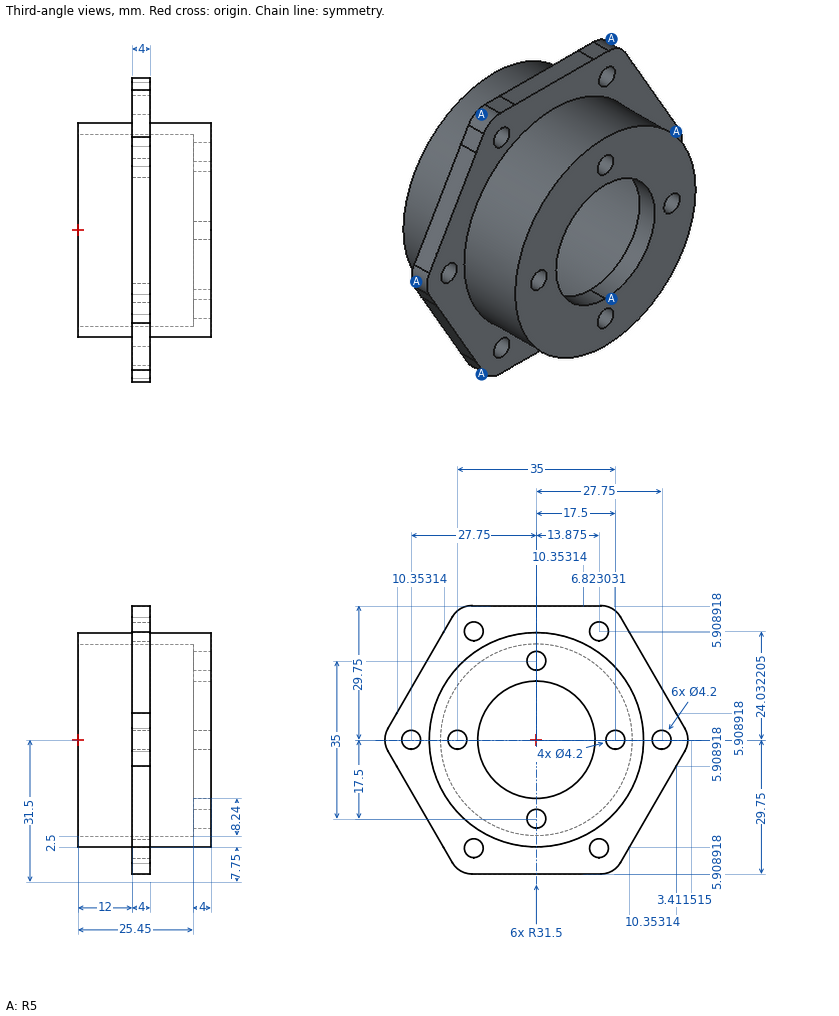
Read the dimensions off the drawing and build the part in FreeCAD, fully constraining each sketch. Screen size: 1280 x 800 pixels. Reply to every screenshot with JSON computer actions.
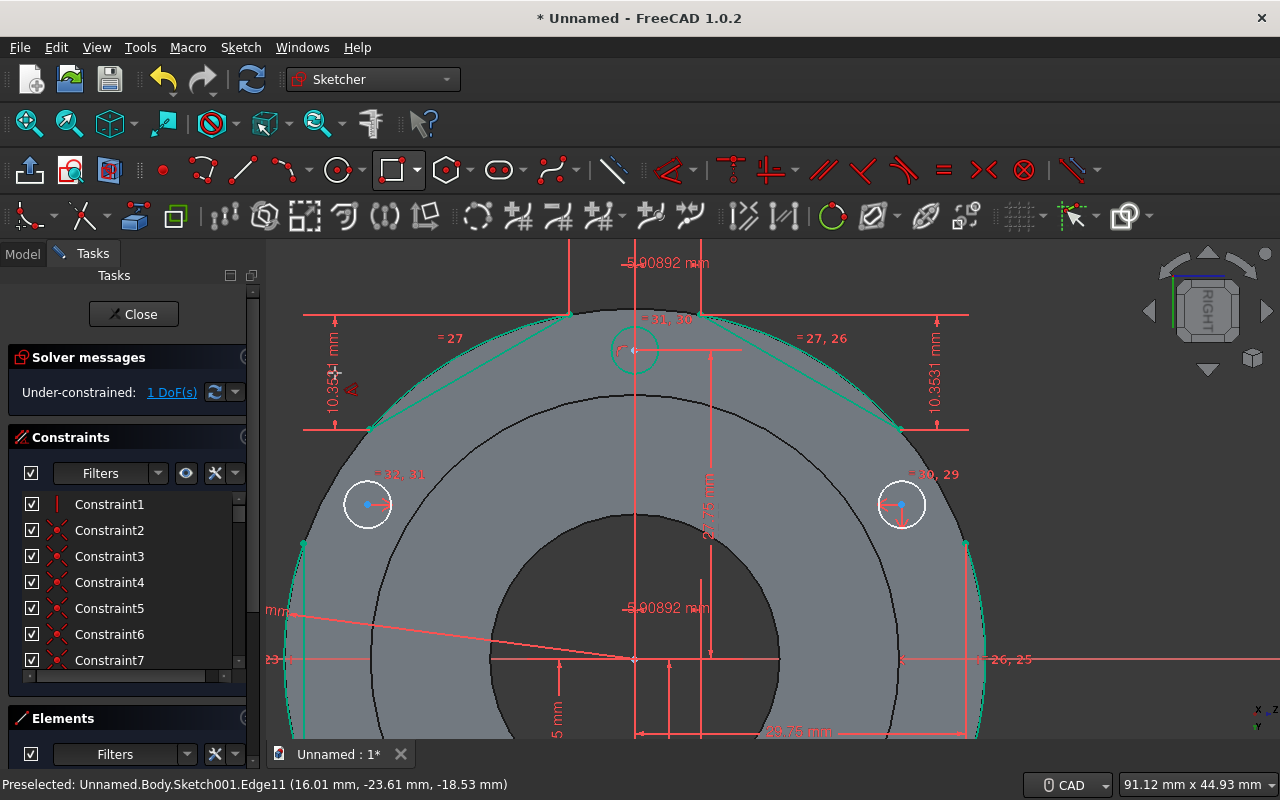
{"action": "scroll", "coordinate": [761, 350], "scroll_direction": "down", "scroll_amount": 4}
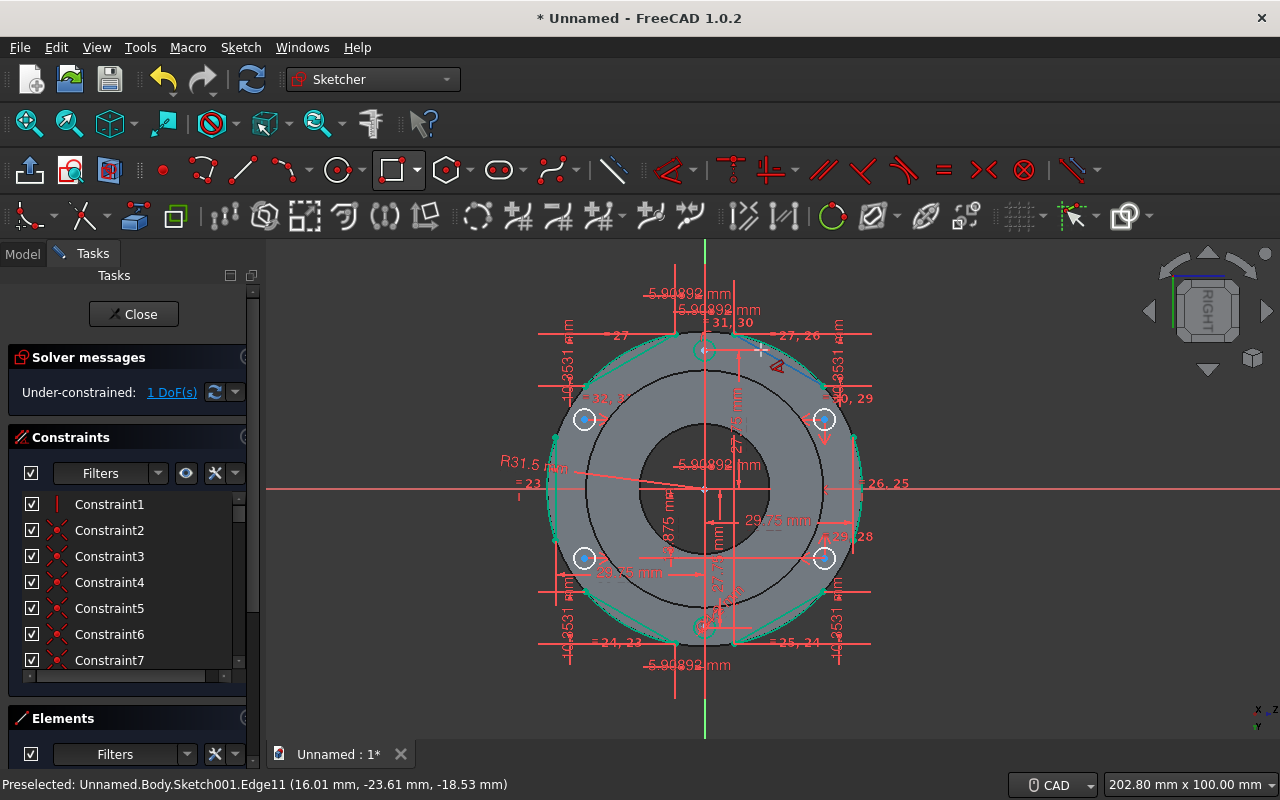
{"action": "left_click", "coordinate": [825, 558]}
{"action": "left_click", "coordinate": [792, 592]}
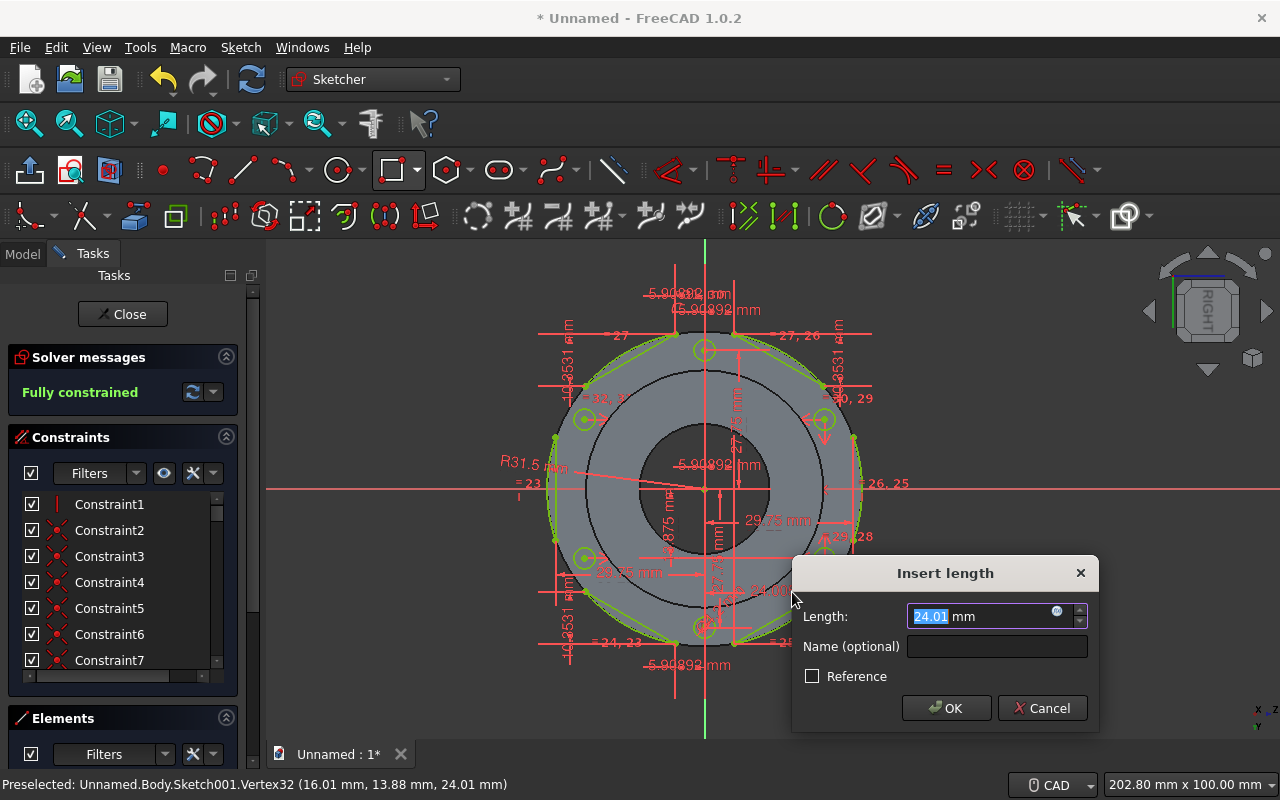
{"action": "type", "text": "24.032205"}
{"action": "key", "text": "Return"}
{"action": "key", "text": "Escape"}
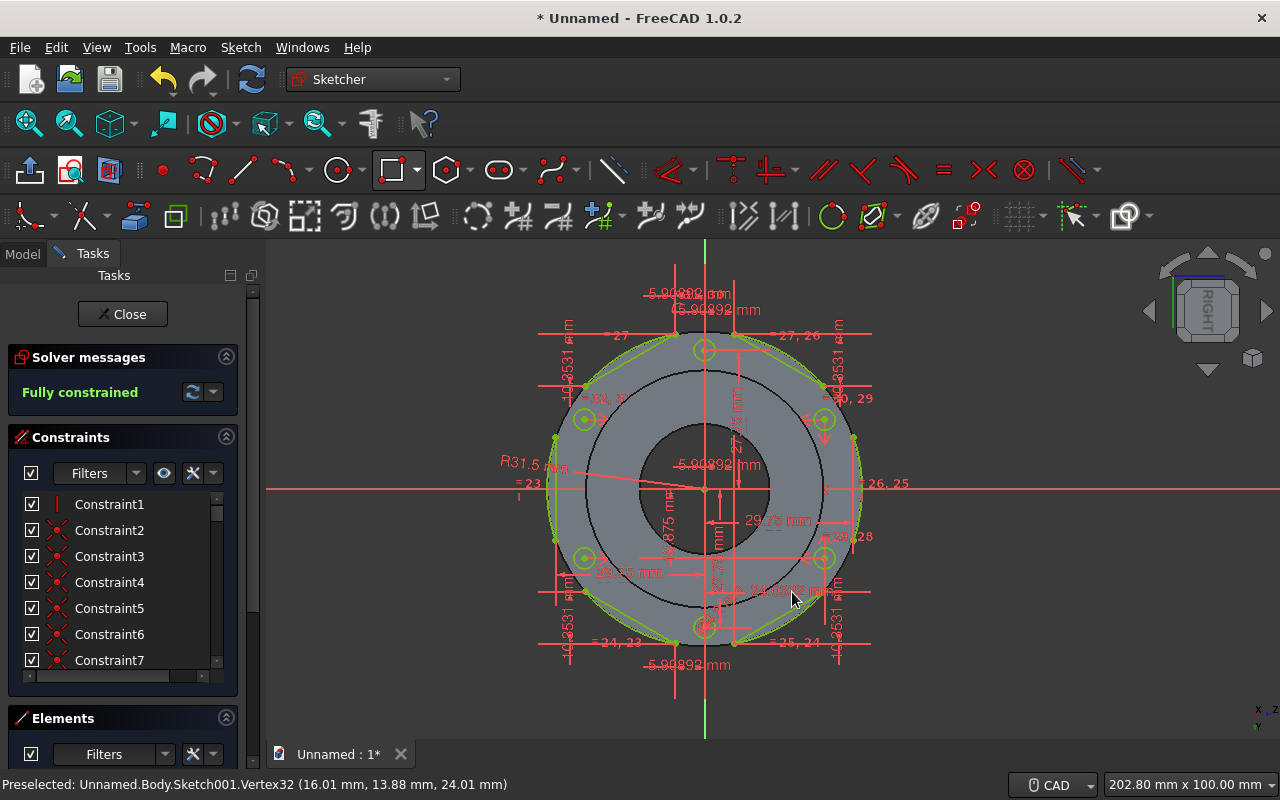
{"action": "left_click", "coordinate": [123, 314]}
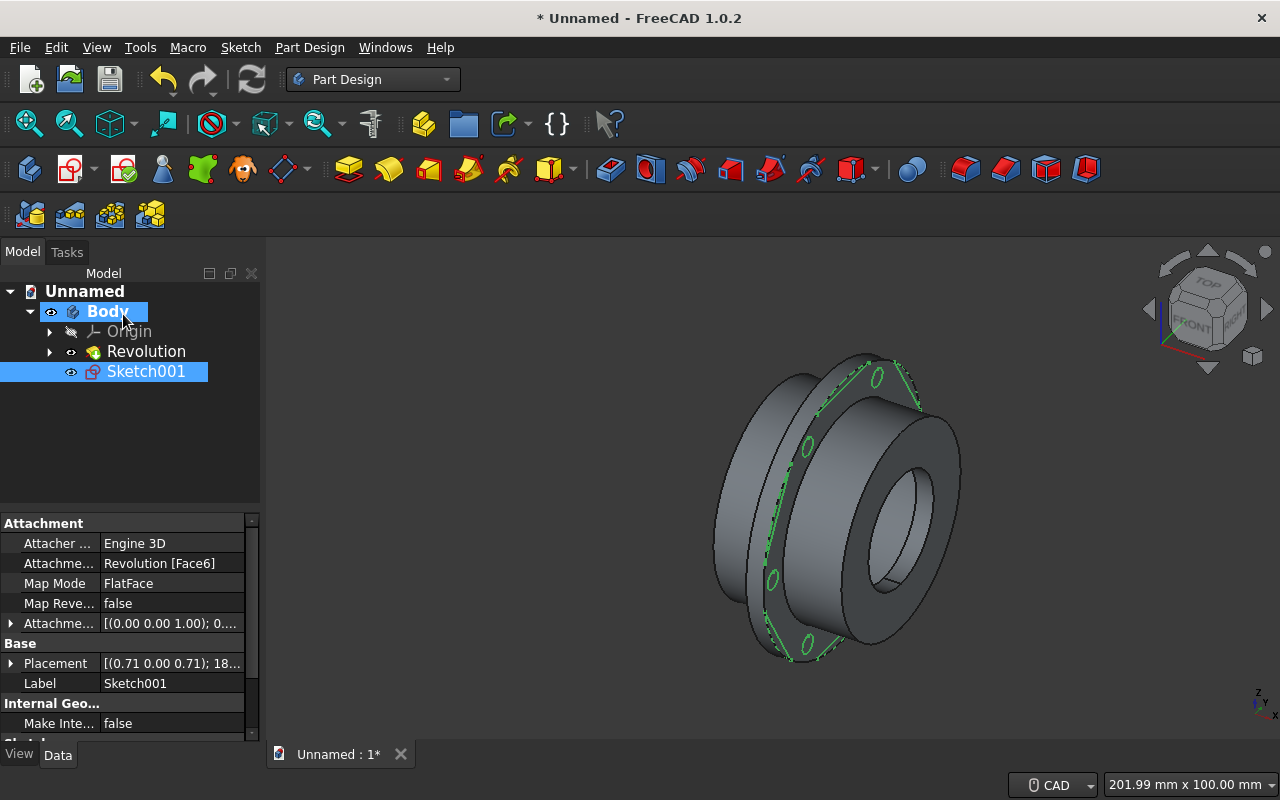
{"action": "left_click", "coordinate": [612, 170]}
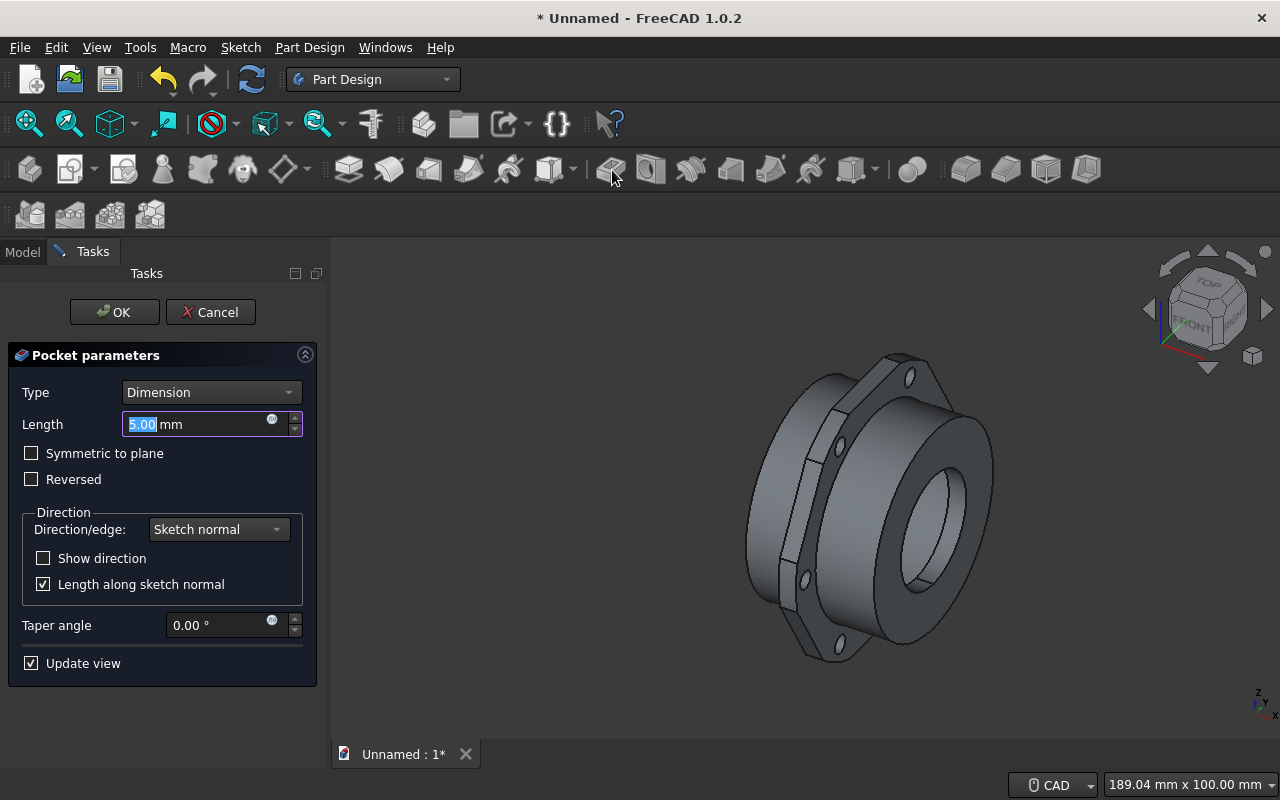
{"action": "left_click", "coordinate": [212, 392]}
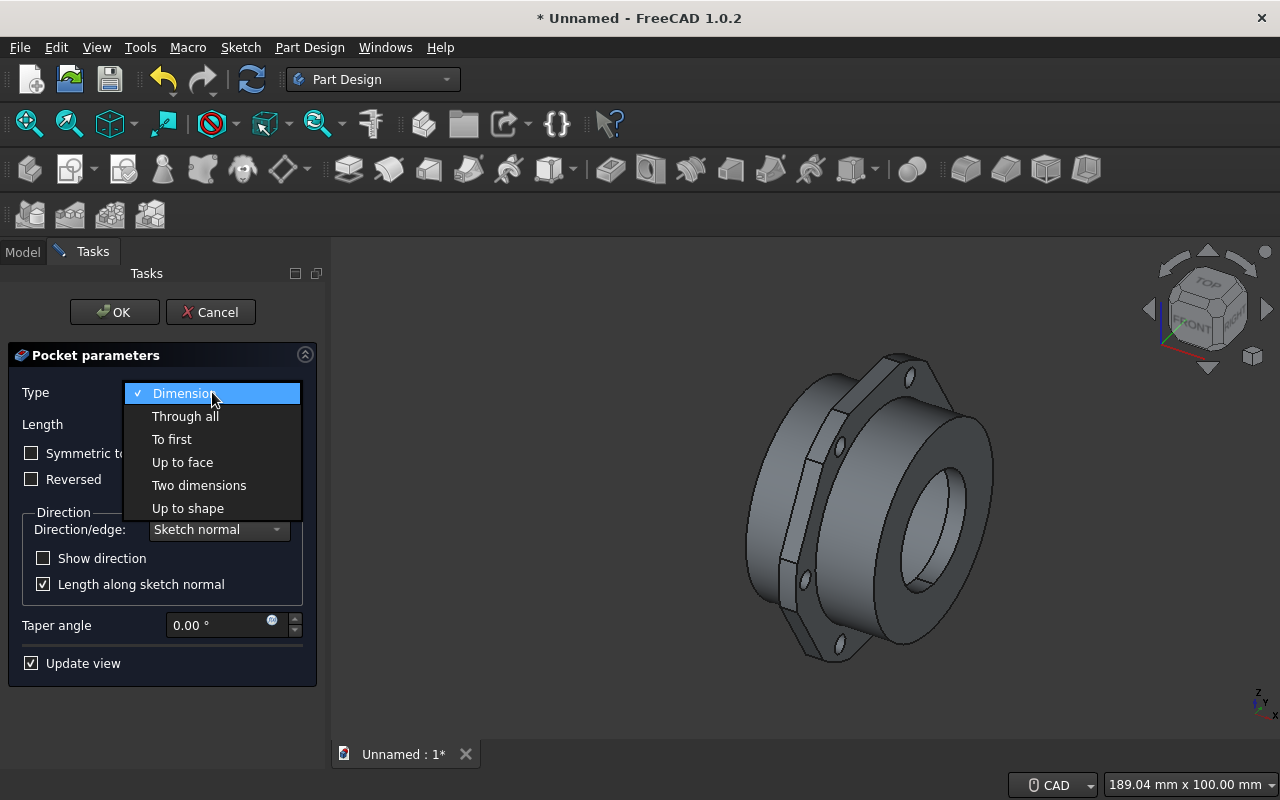
{"action": "left_click", "coordinate": [212, 416]}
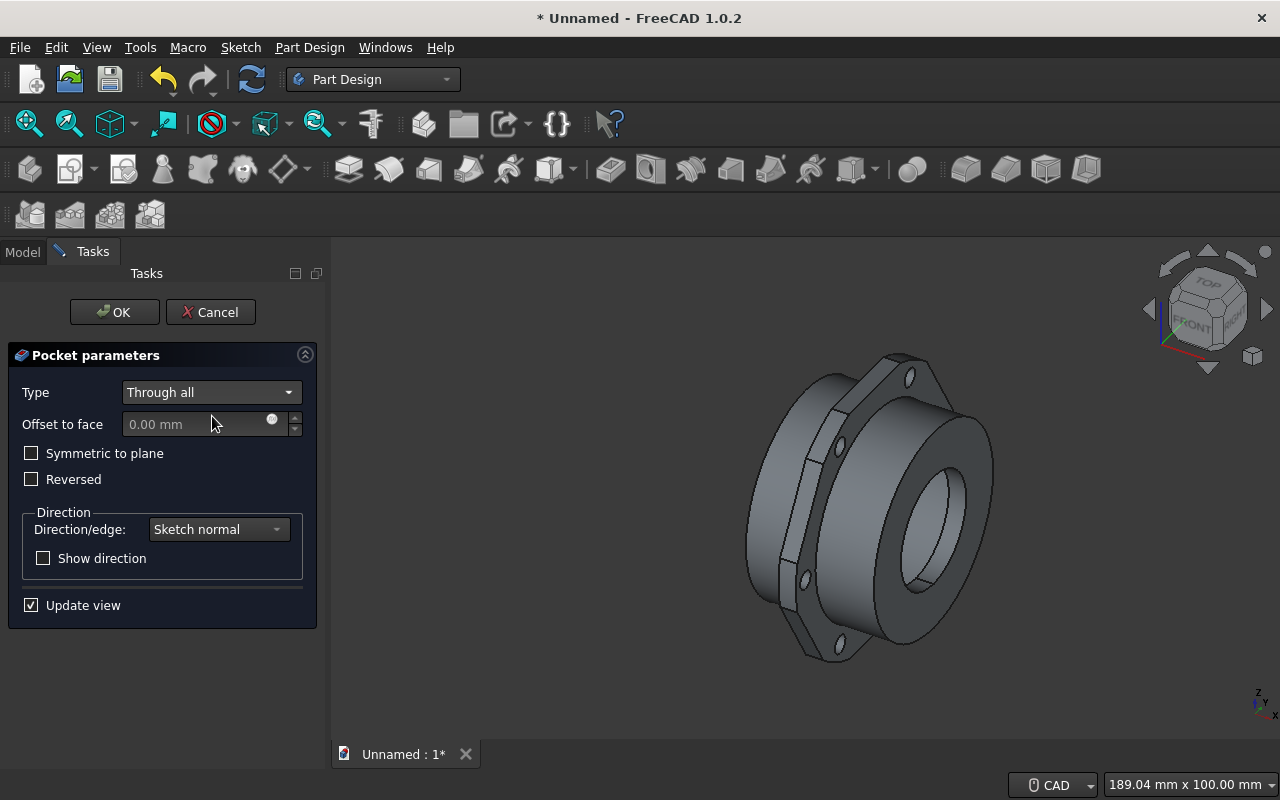
{"action": "left_click", "coordinate": [115, 312]}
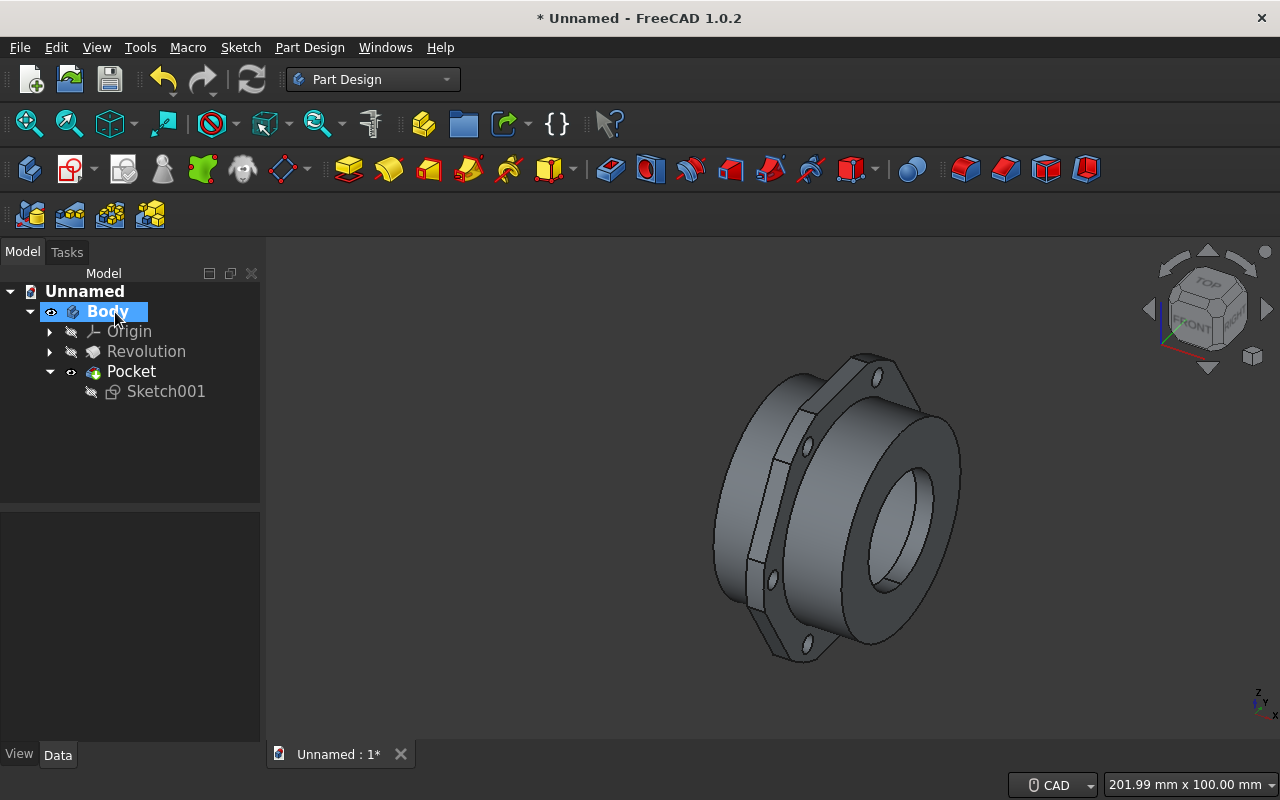
{"action": "left_click", "coordinate": [935, 440]}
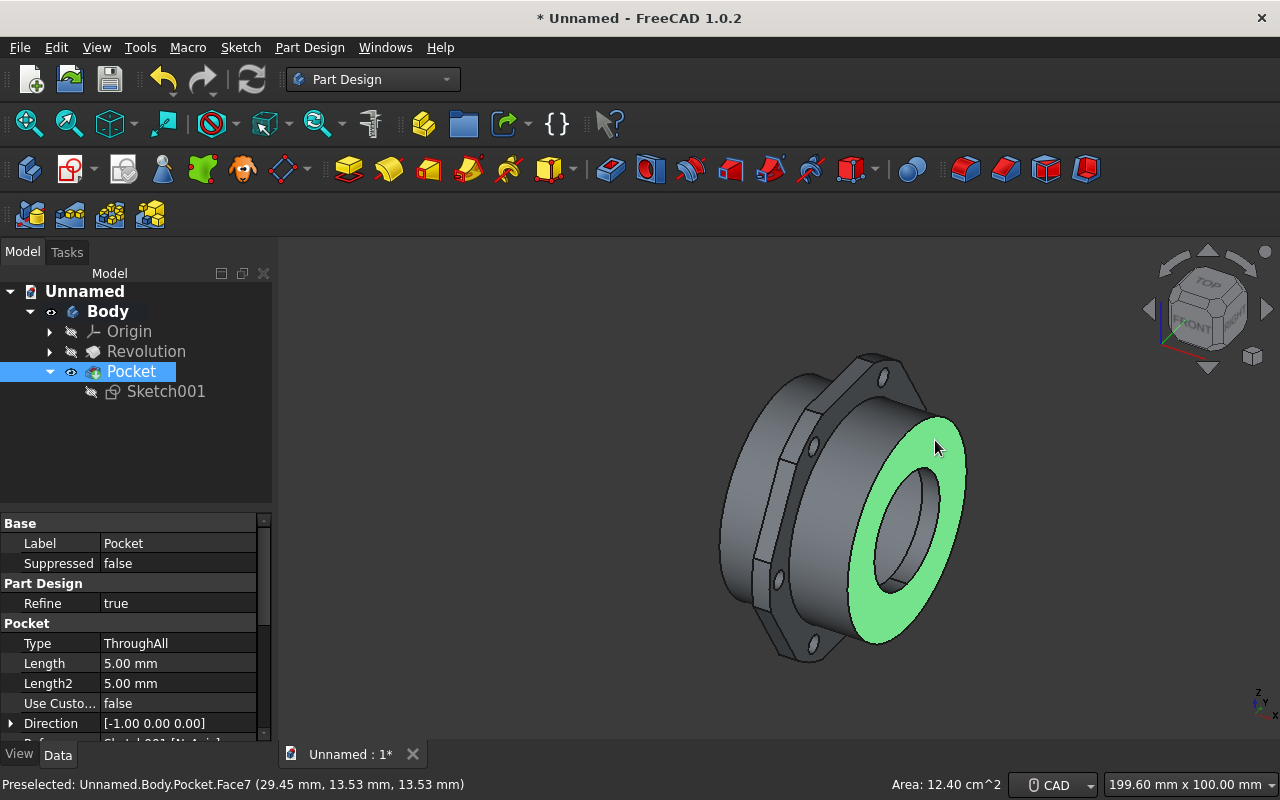
{"action": "left_click", "coordinate": [70, 170]}